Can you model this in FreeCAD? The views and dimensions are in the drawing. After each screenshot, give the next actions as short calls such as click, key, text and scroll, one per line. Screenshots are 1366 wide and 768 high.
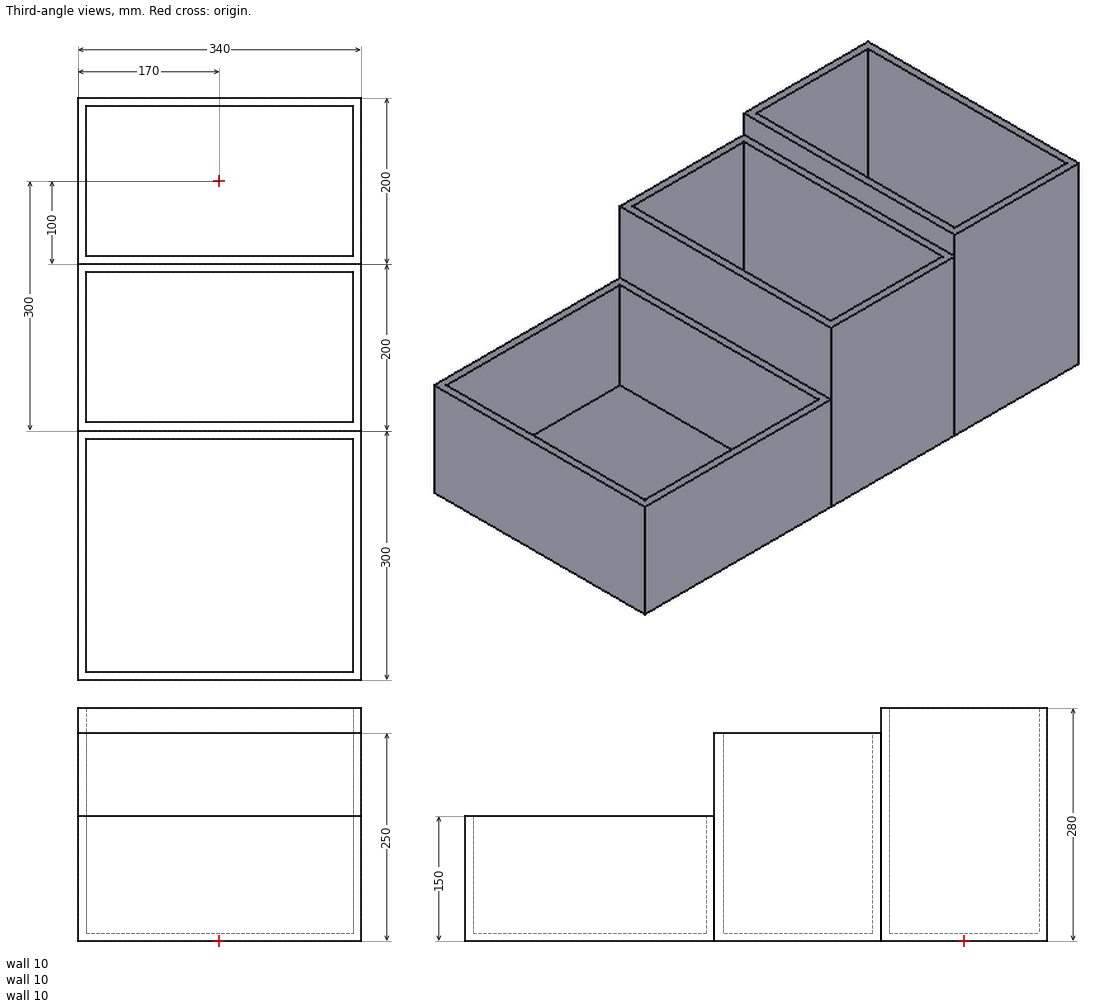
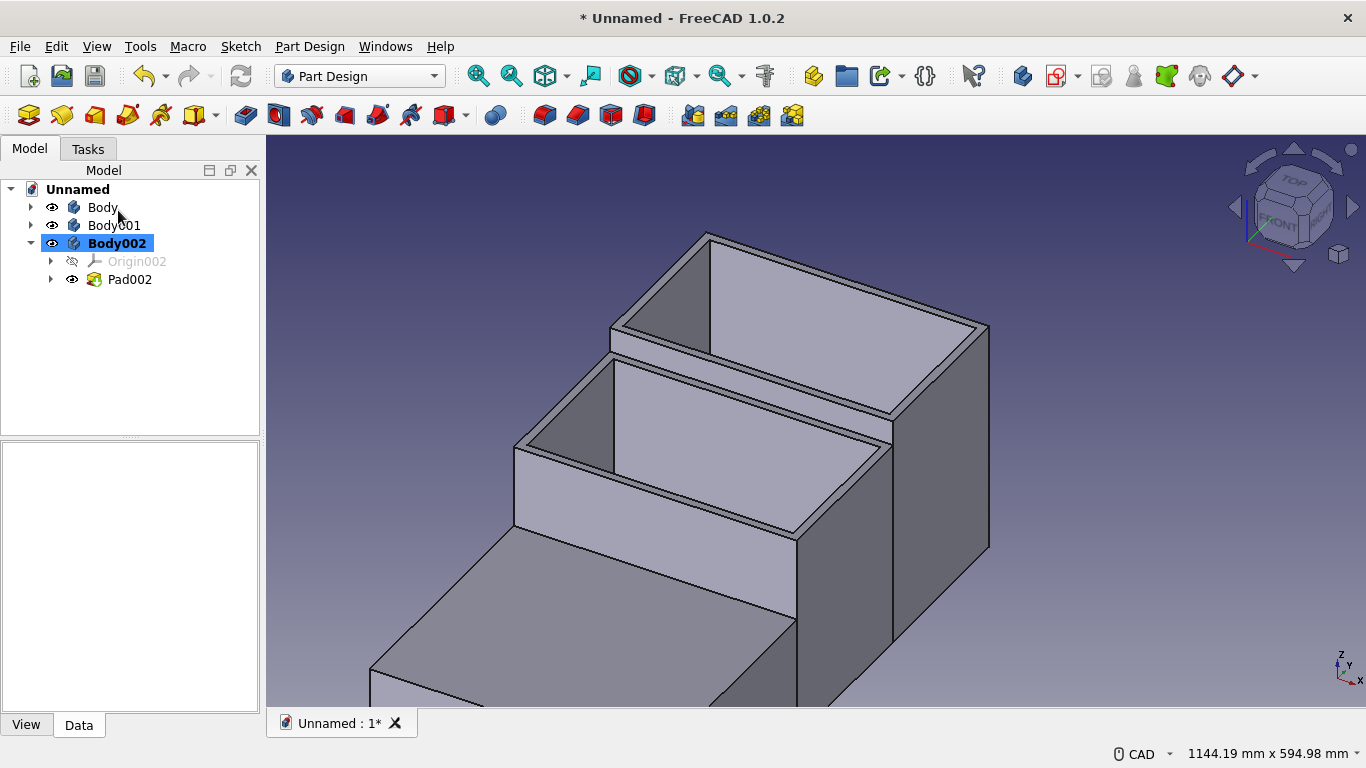
click(479, 76)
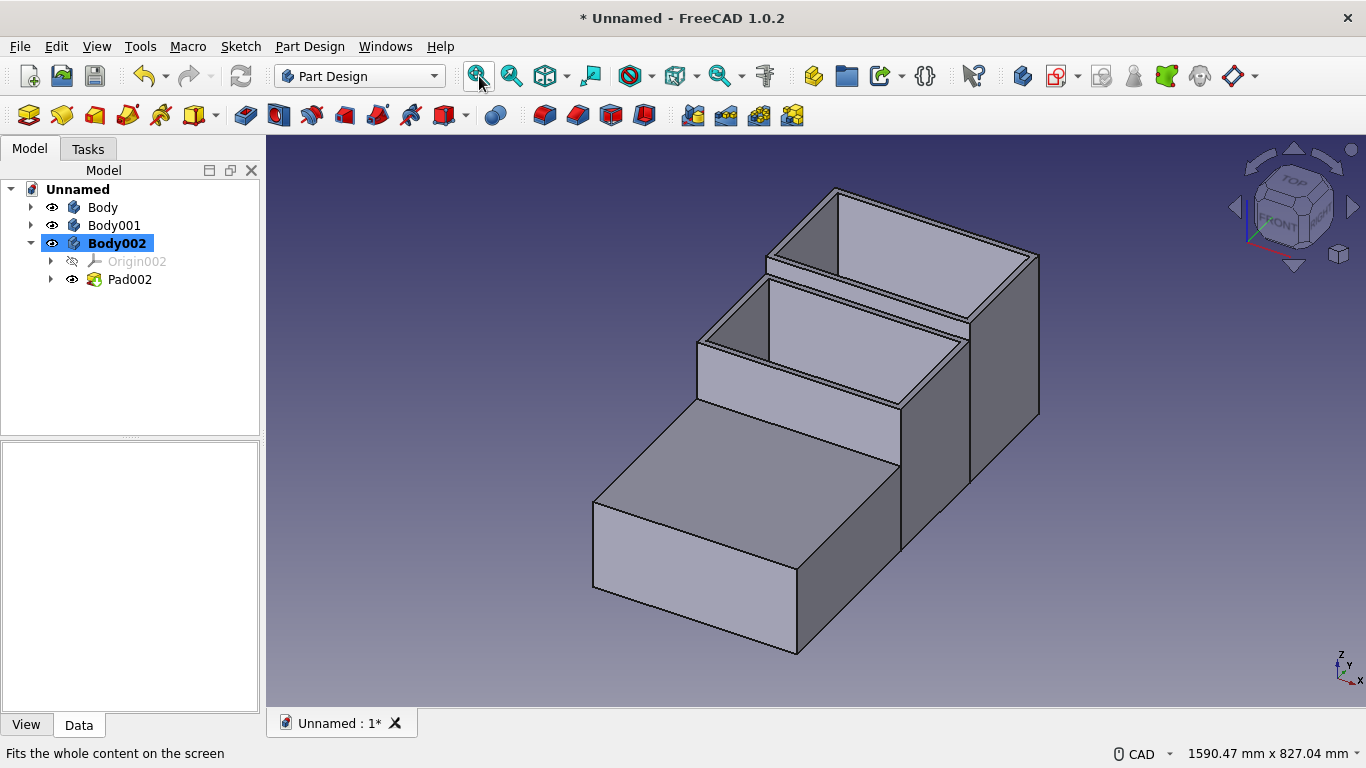
click(747, 483)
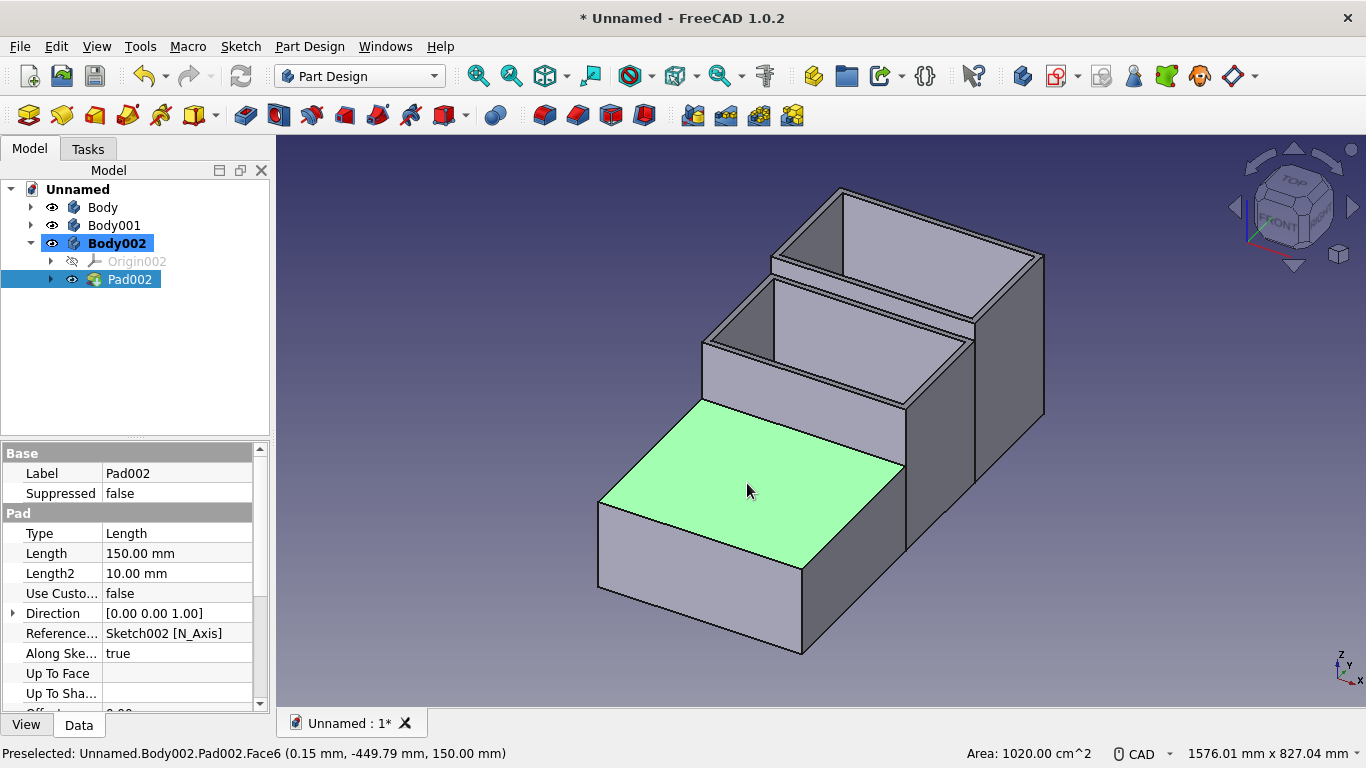
click(644, 116)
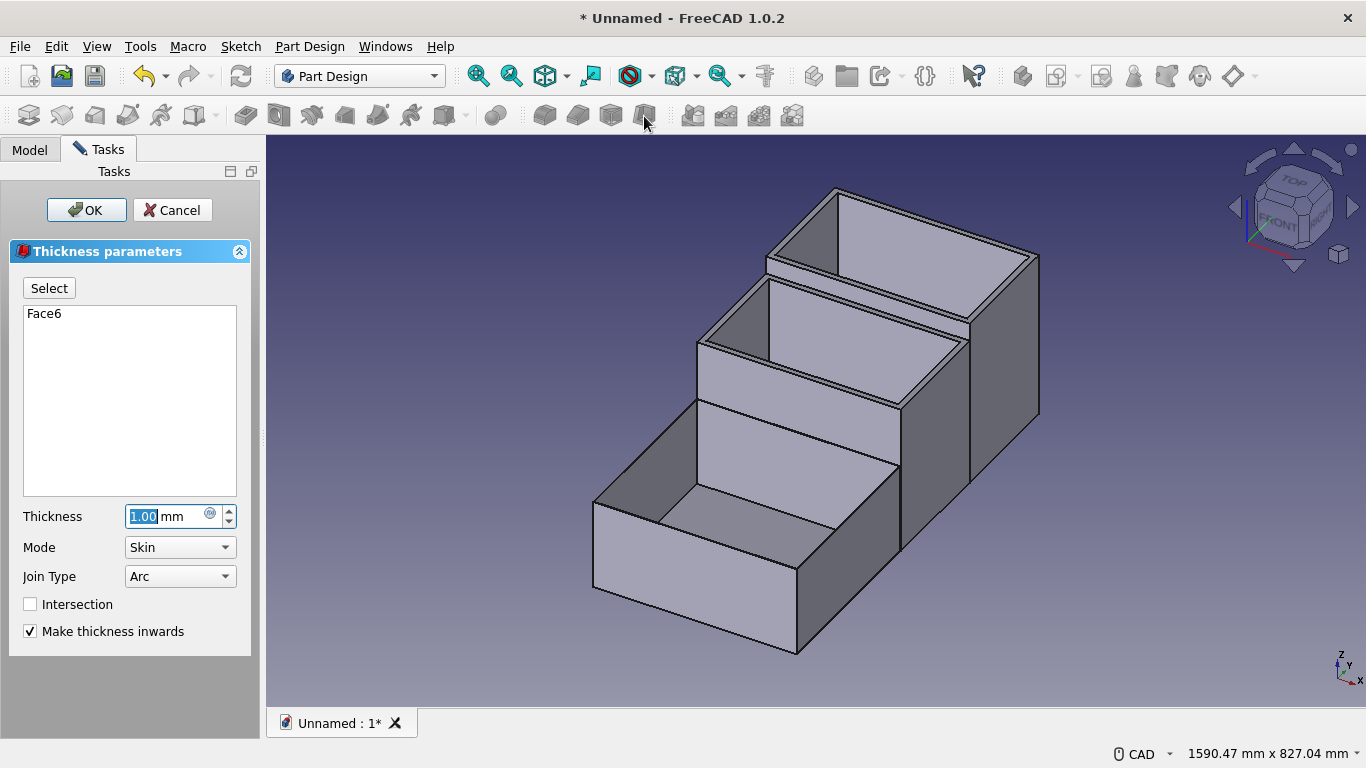
text(10)
key(Tab)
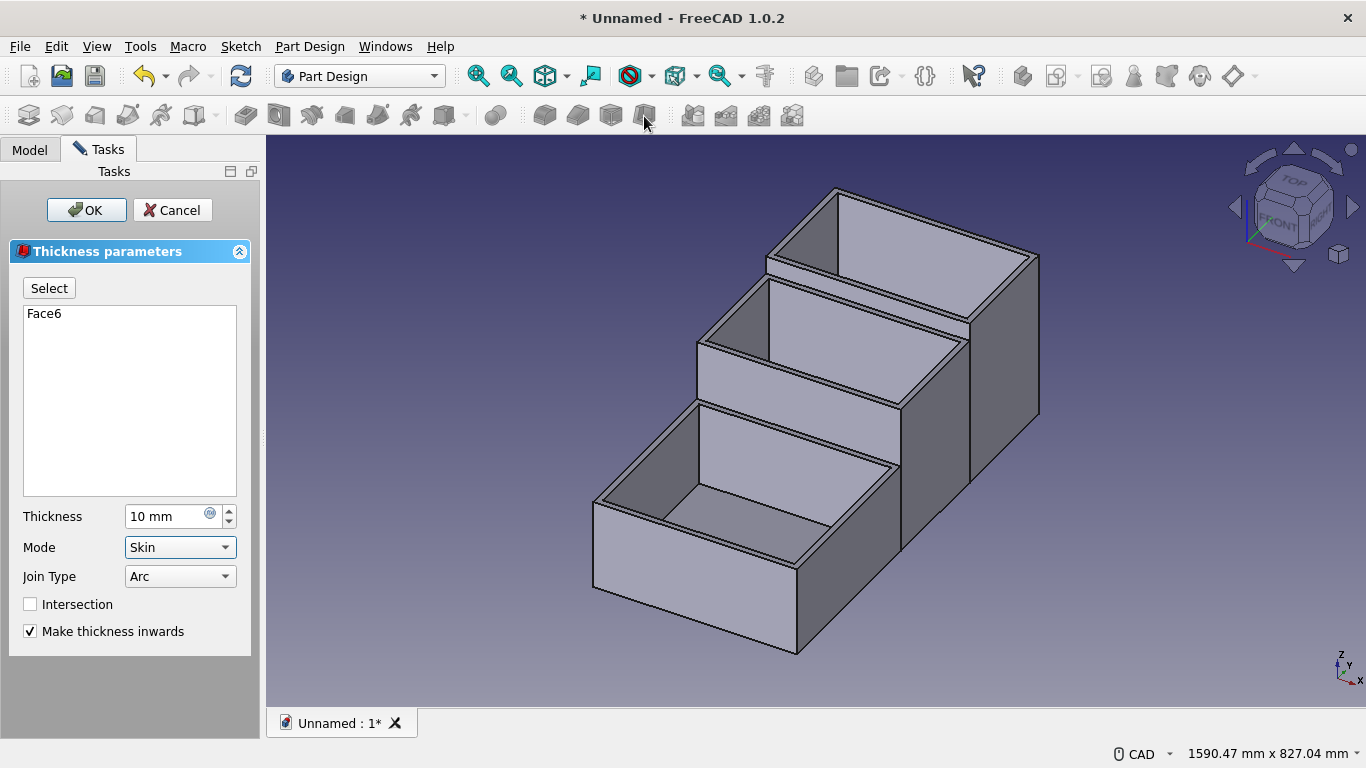
click(181, 576)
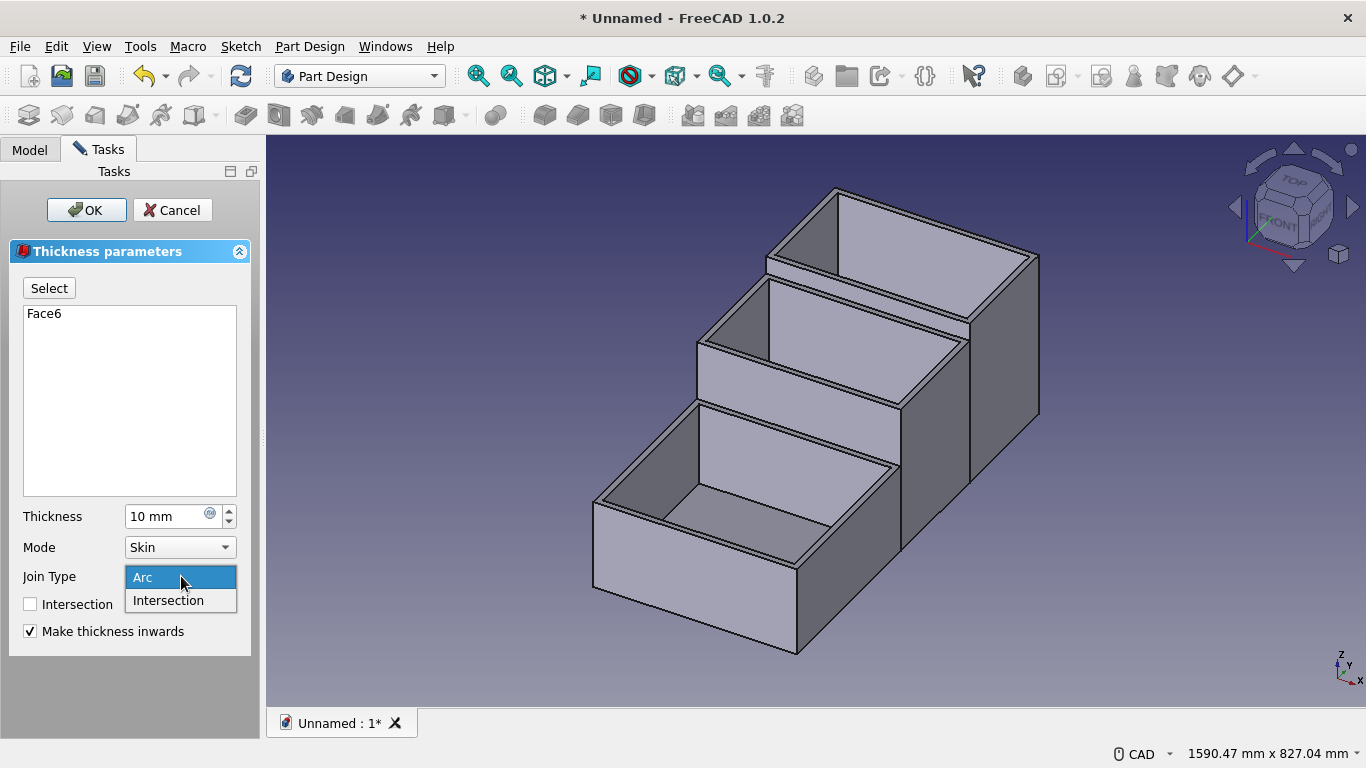
click(179, 600)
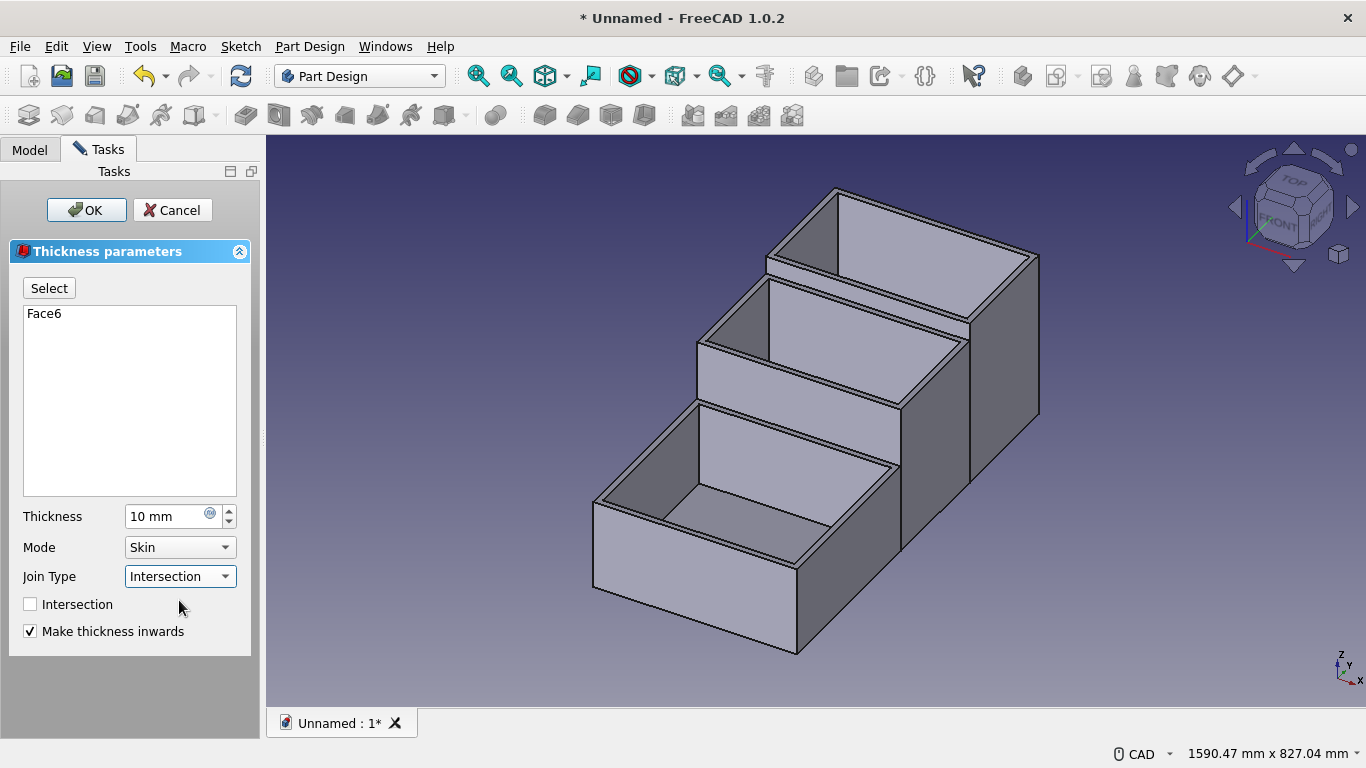
click(87, 210)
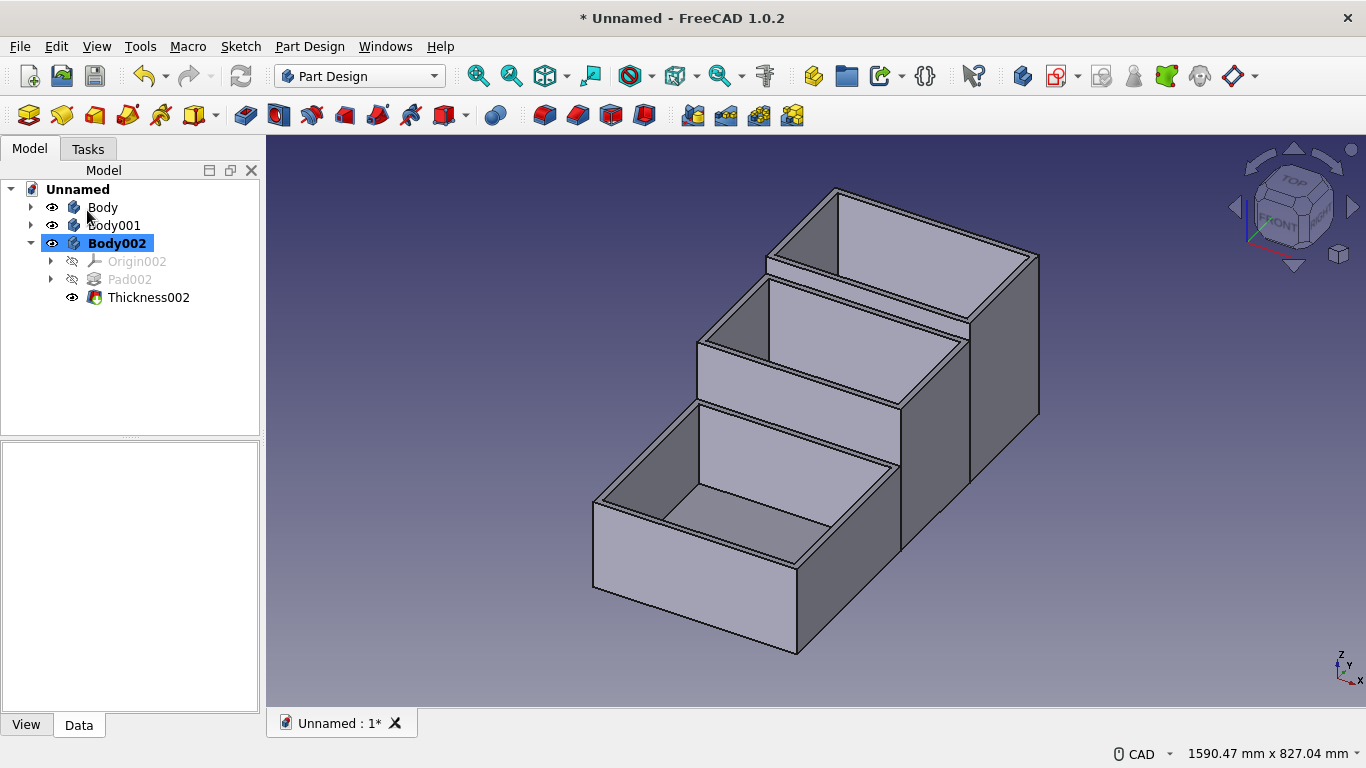
key(0)